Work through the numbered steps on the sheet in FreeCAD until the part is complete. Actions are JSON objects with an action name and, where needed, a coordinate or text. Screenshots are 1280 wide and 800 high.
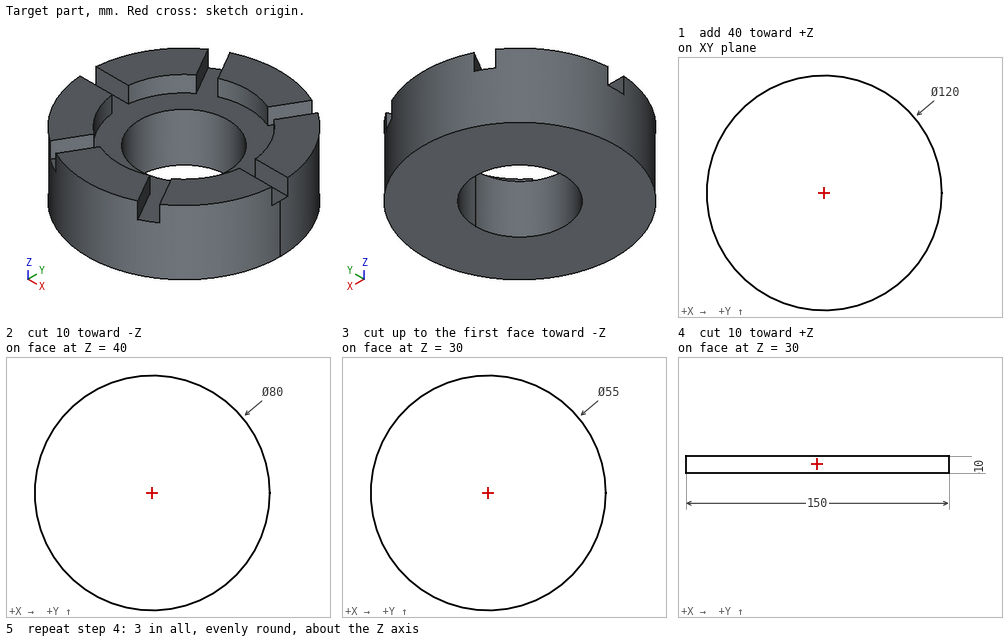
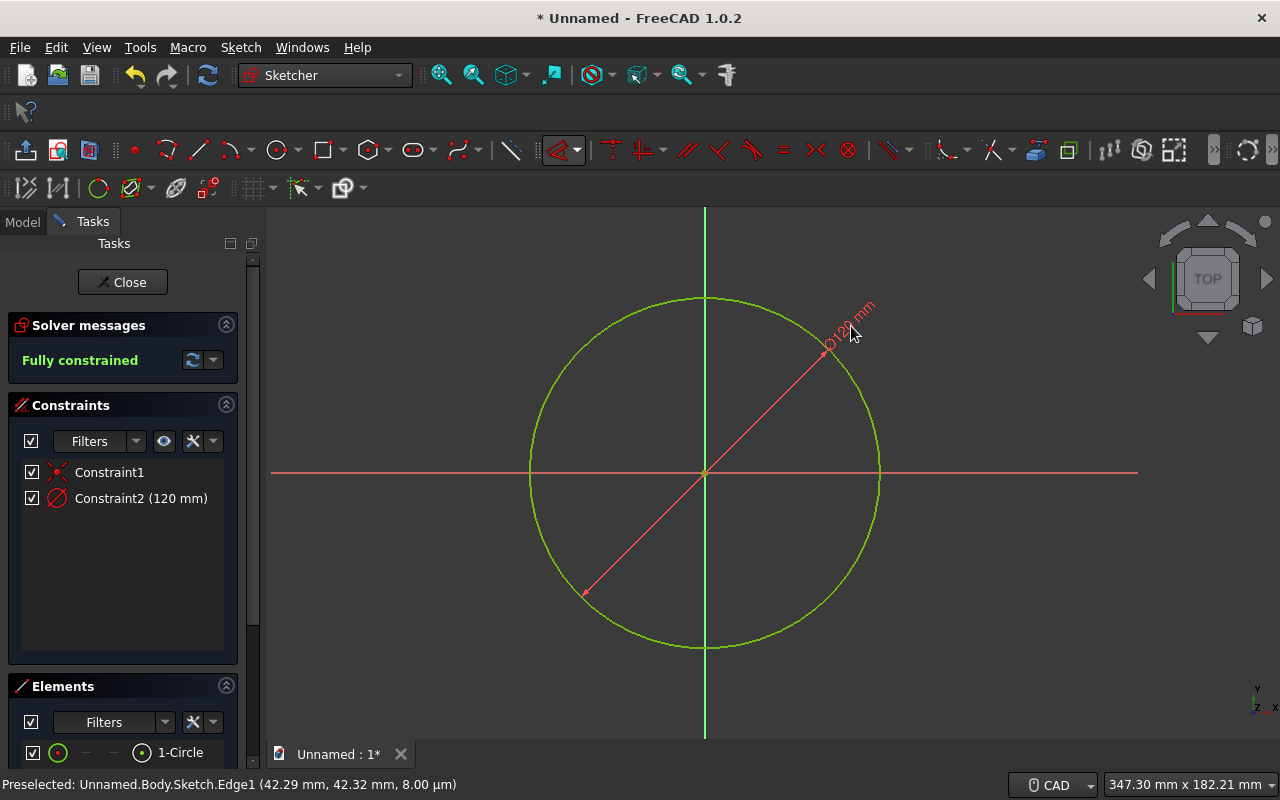
{"action": "left_click", "coordinate": [123, 282]}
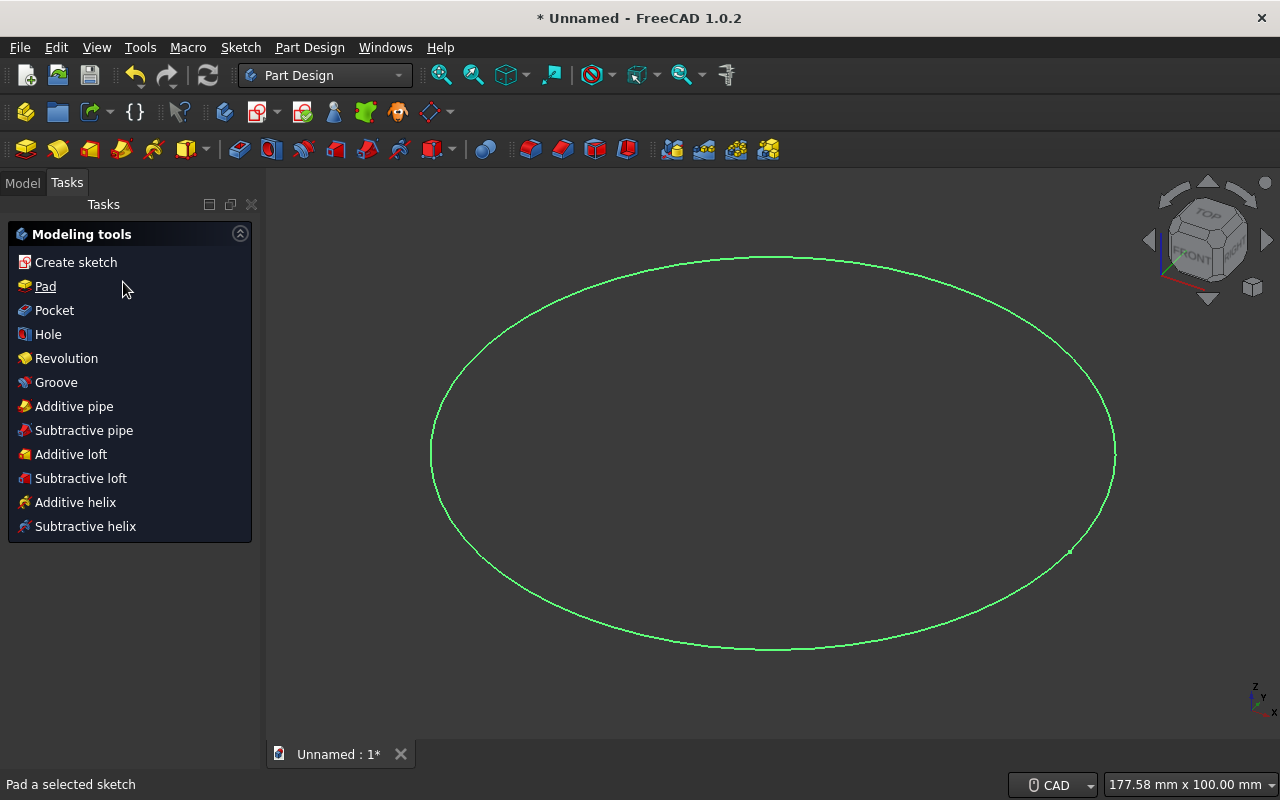
{"action": "left_click", "coordinate": [26, 150]}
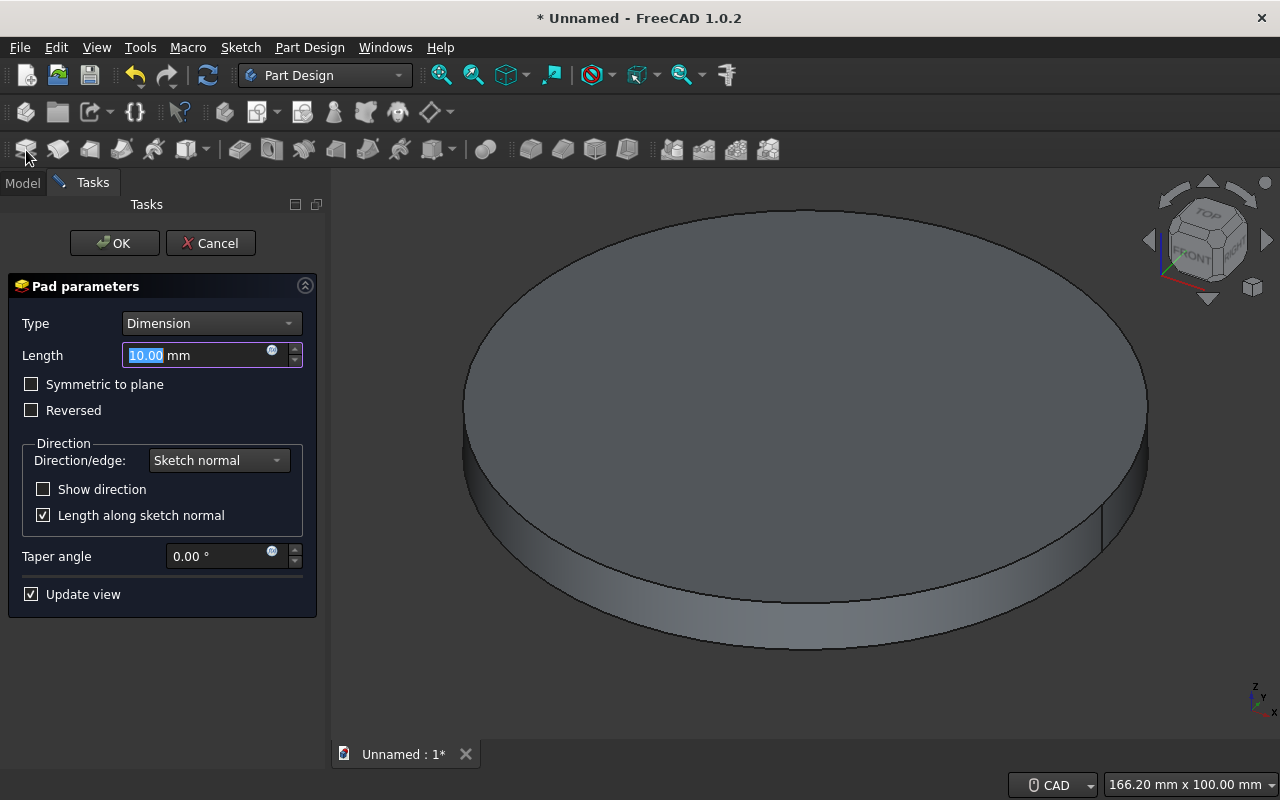
{"action": "type", "text": "40"}
{"action": "key", "text": "Tab"}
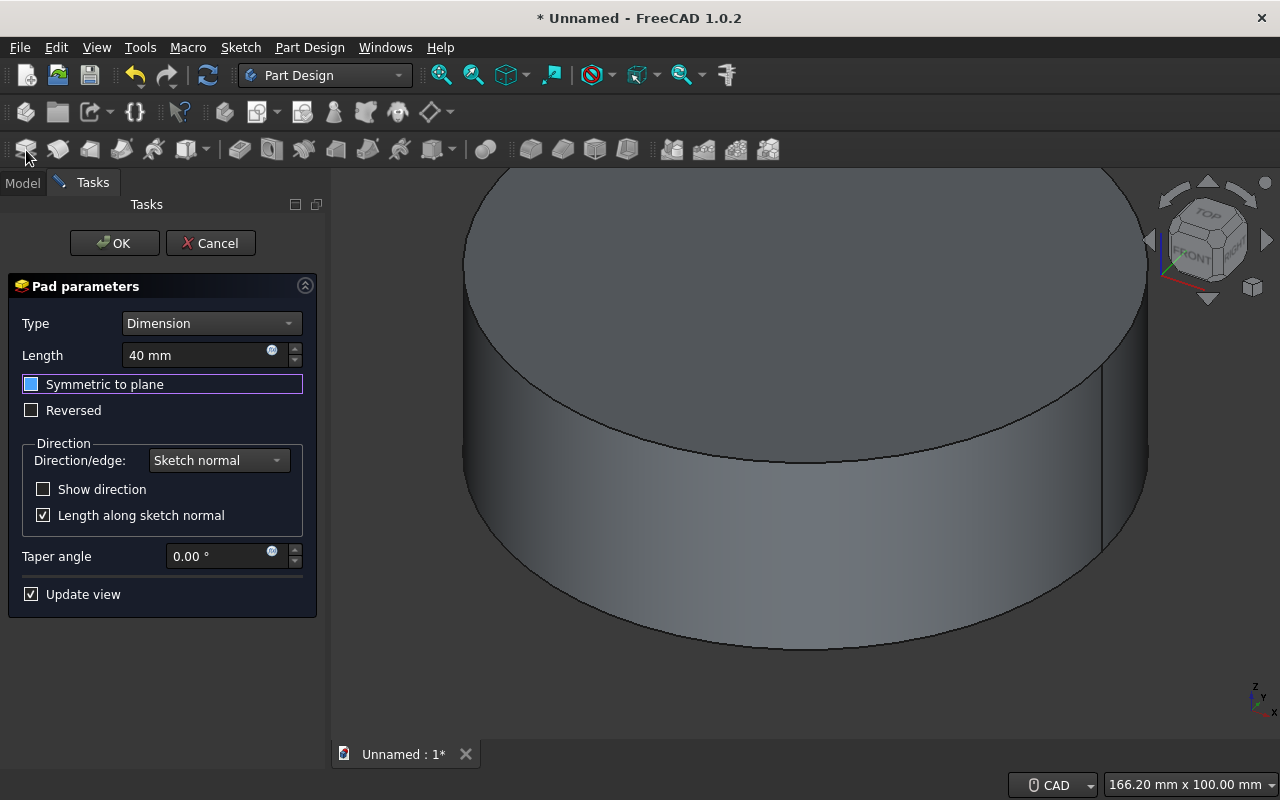
{"action": "left_click", "coordinate": [115, 243]}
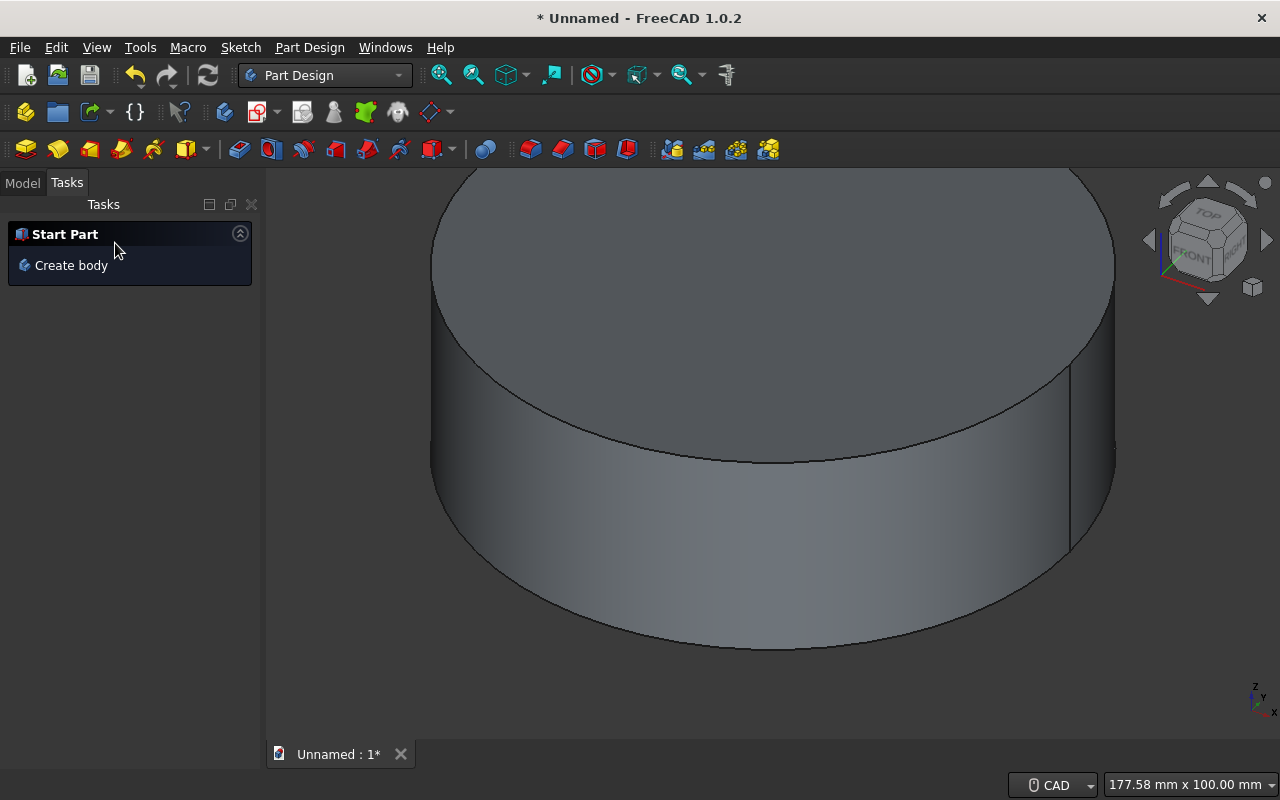
{"action": "left_click", "coordinate": [442, 76]}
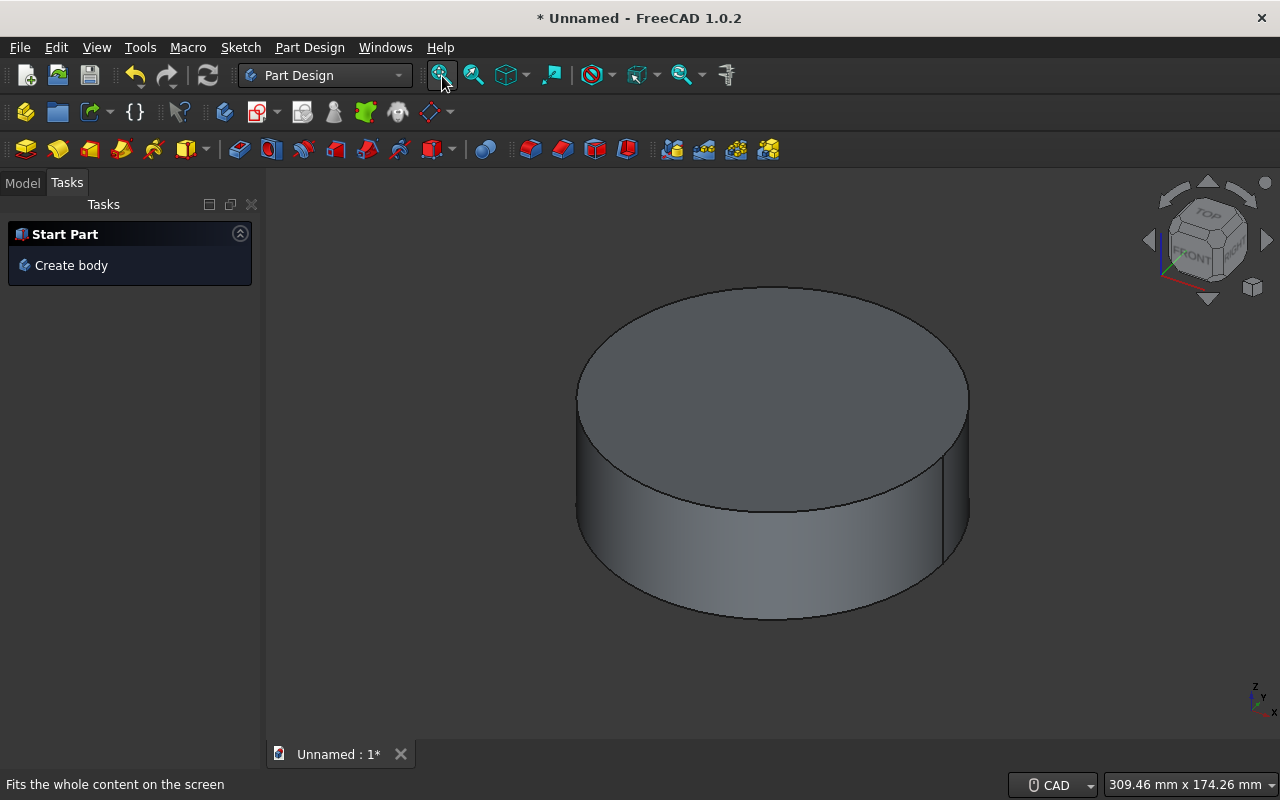
{"action": "left_click", "coordinate": [773, 399]}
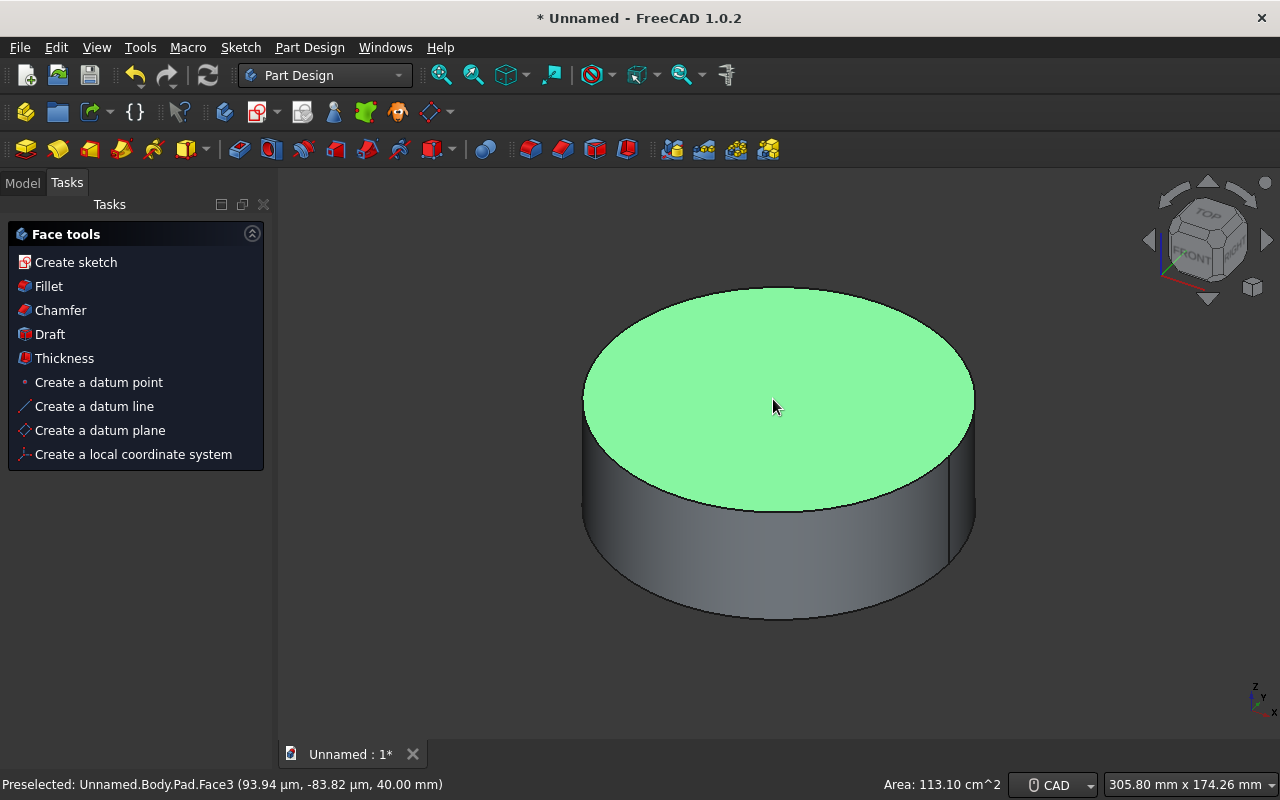
{"action": "left_click", "coordinate": [258, 112]}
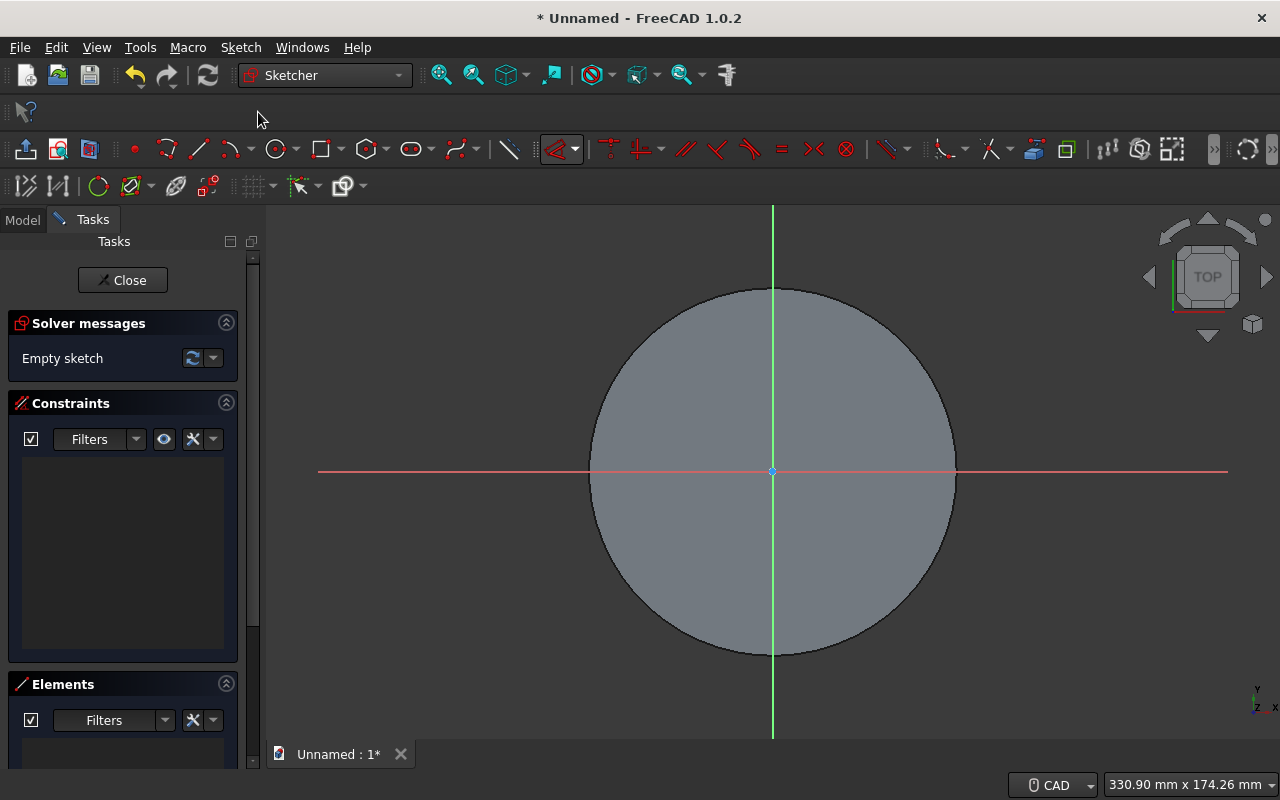
{"action": "scroll", "coordinate": [912, 472], "scroll_direction": "up", "scroll_amount": 2}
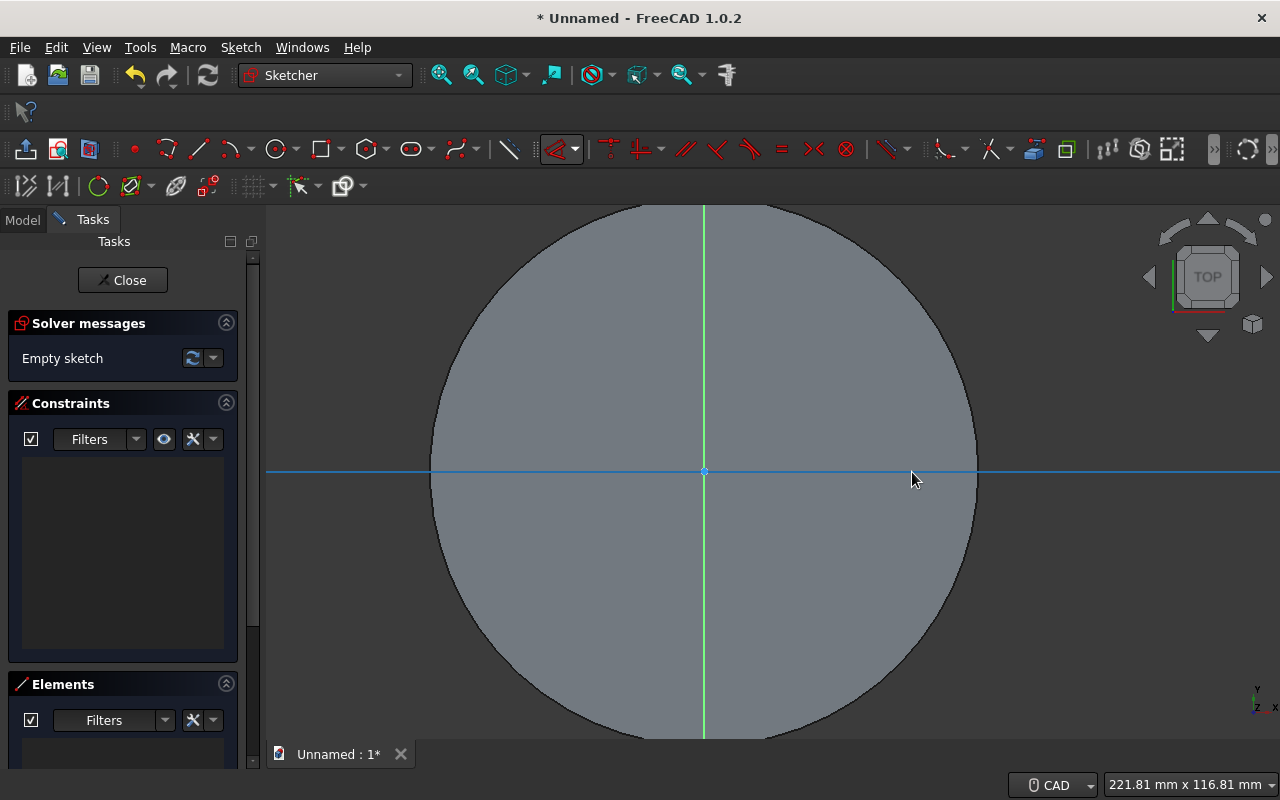
{"action": "key", "text": "g c"}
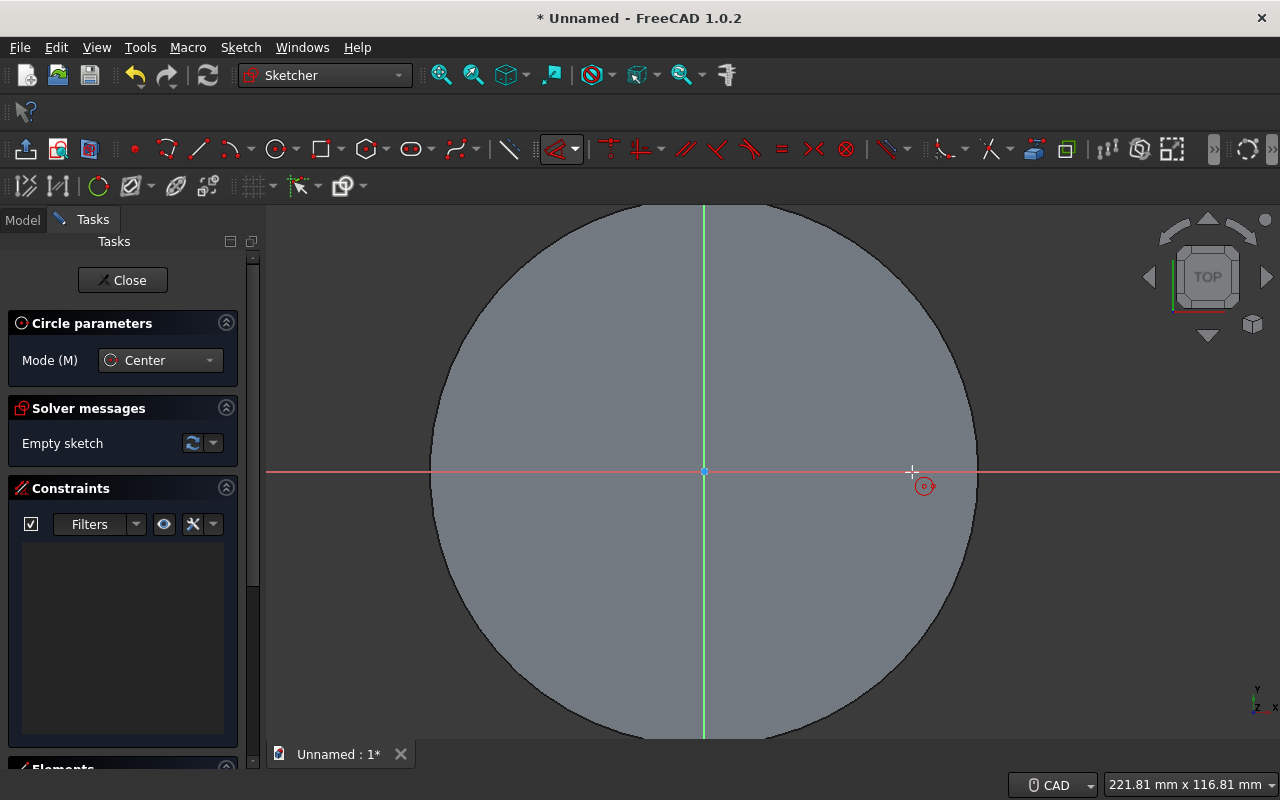
{"action": "left_click", "coordinate": [704, 472]}
{"action": "left_click", "coordinate": [833, 342]}
{"action": "key", "text": "Escape"}